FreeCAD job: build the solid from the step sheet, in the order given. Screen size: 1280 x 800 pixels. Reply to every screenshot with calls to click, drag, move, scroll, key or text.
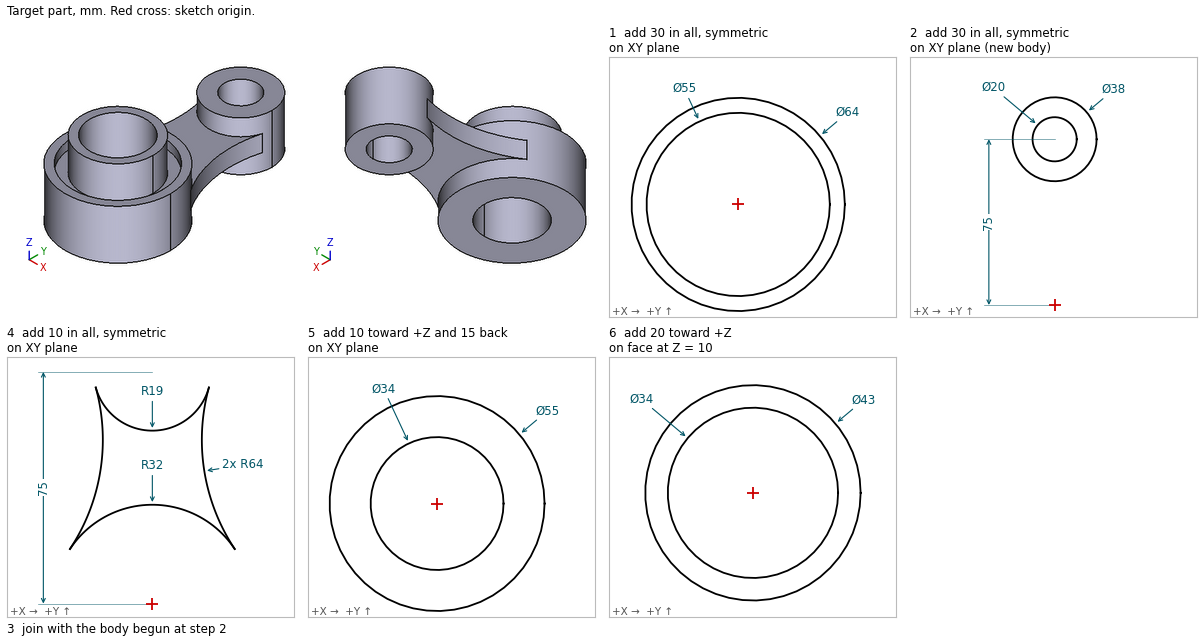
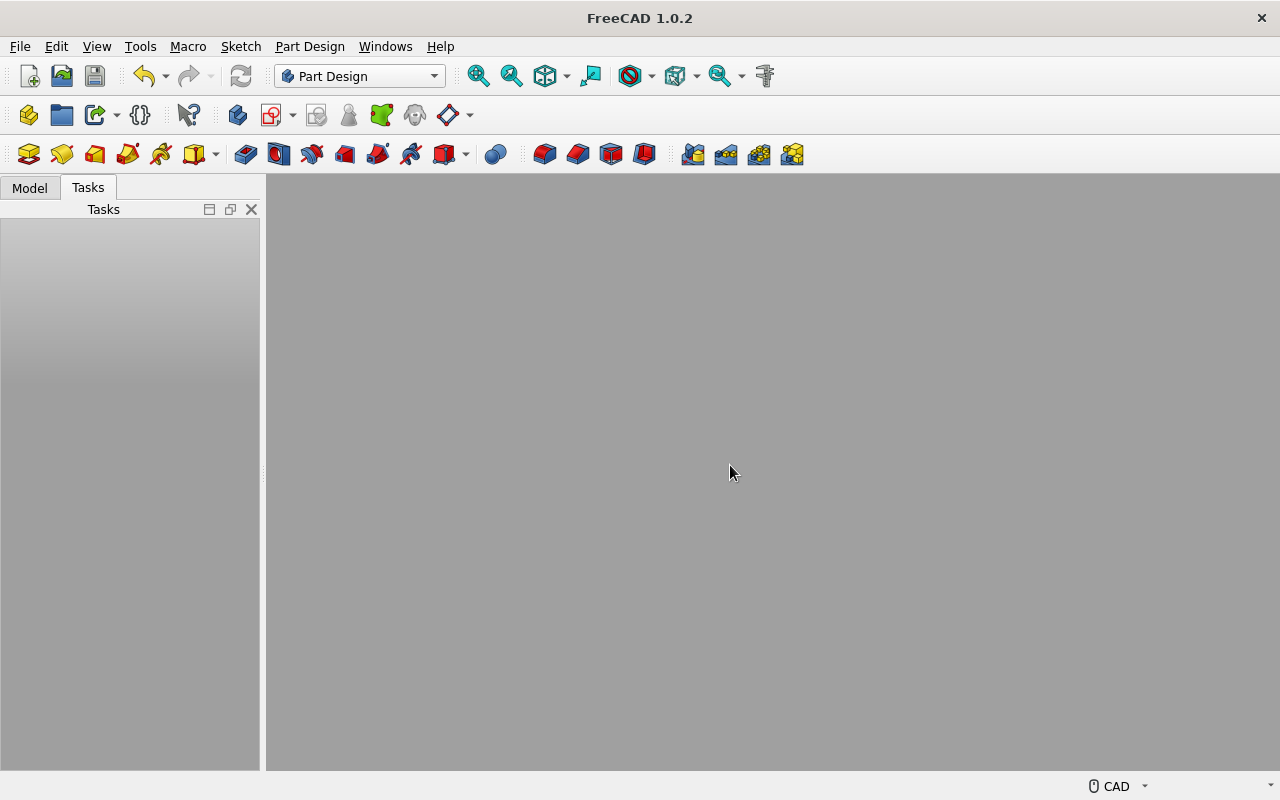
click(29, 76)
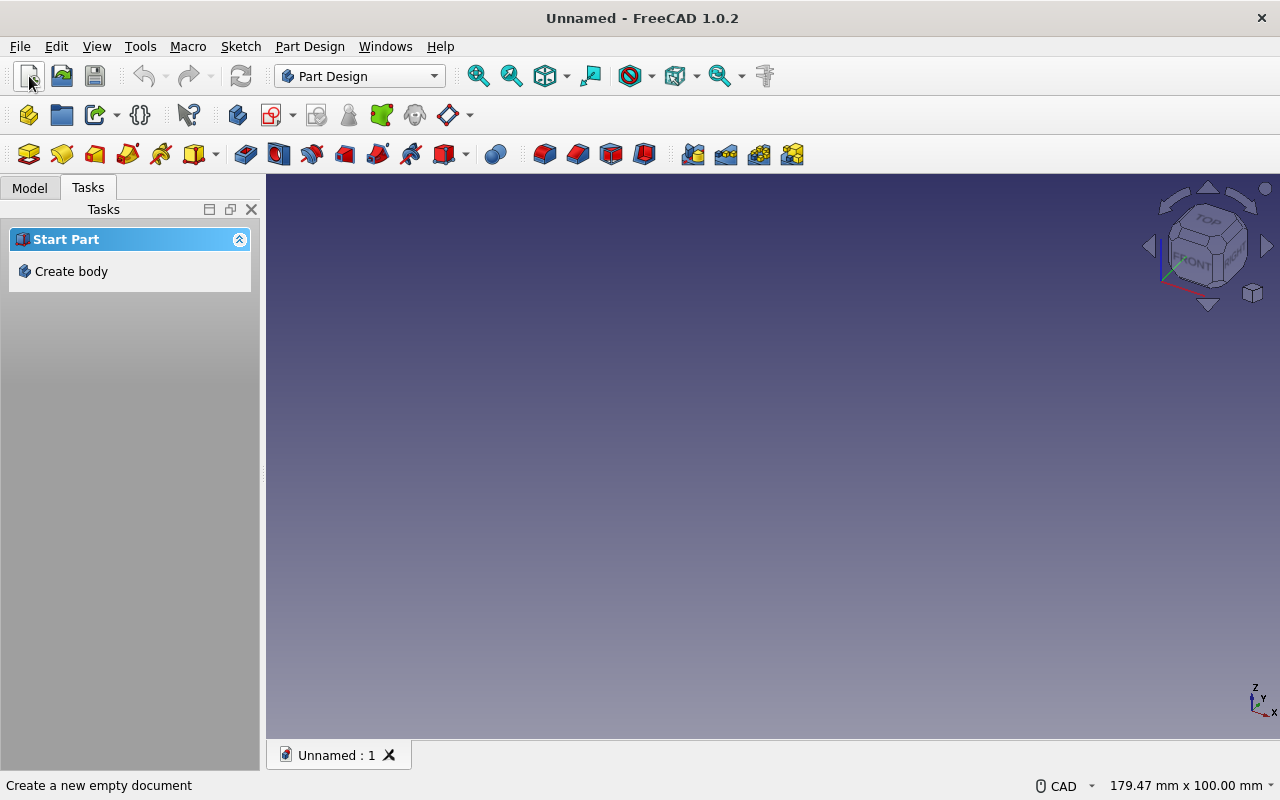
click(270, 116)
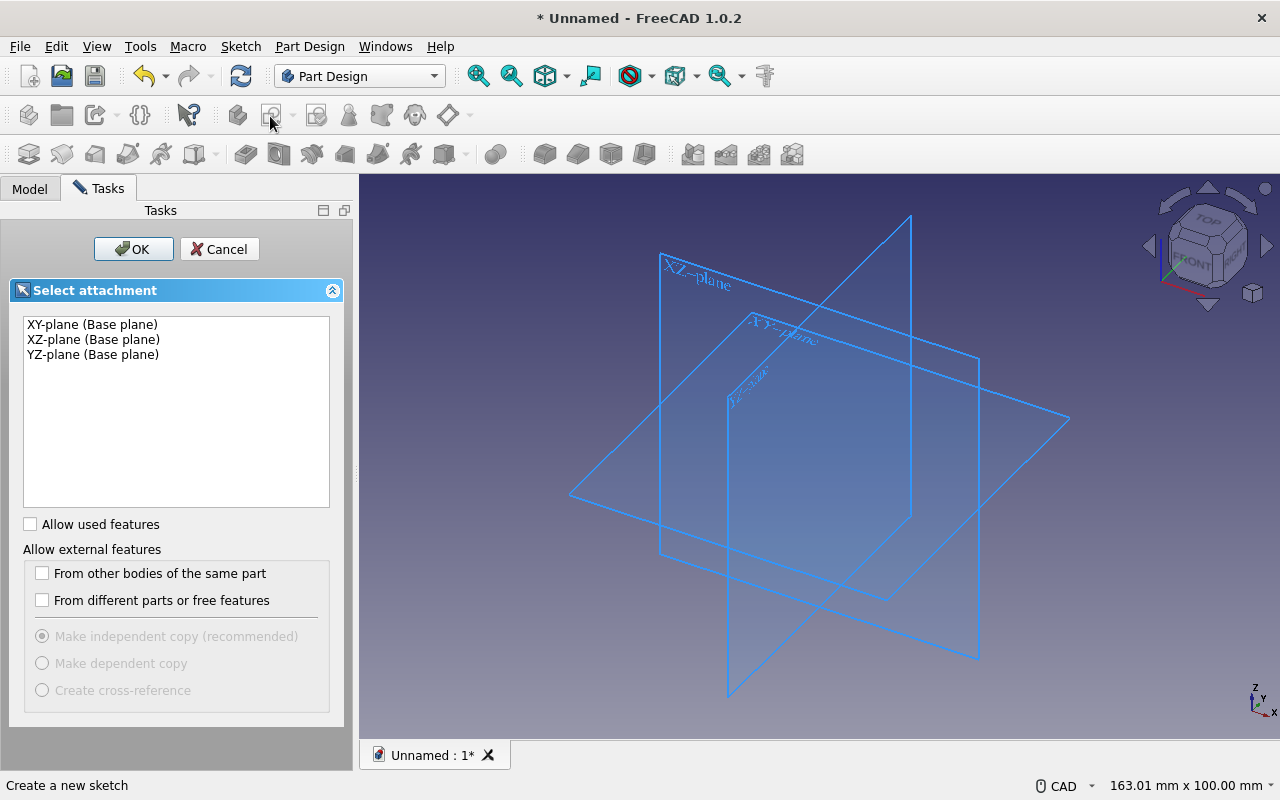
click(84, 324)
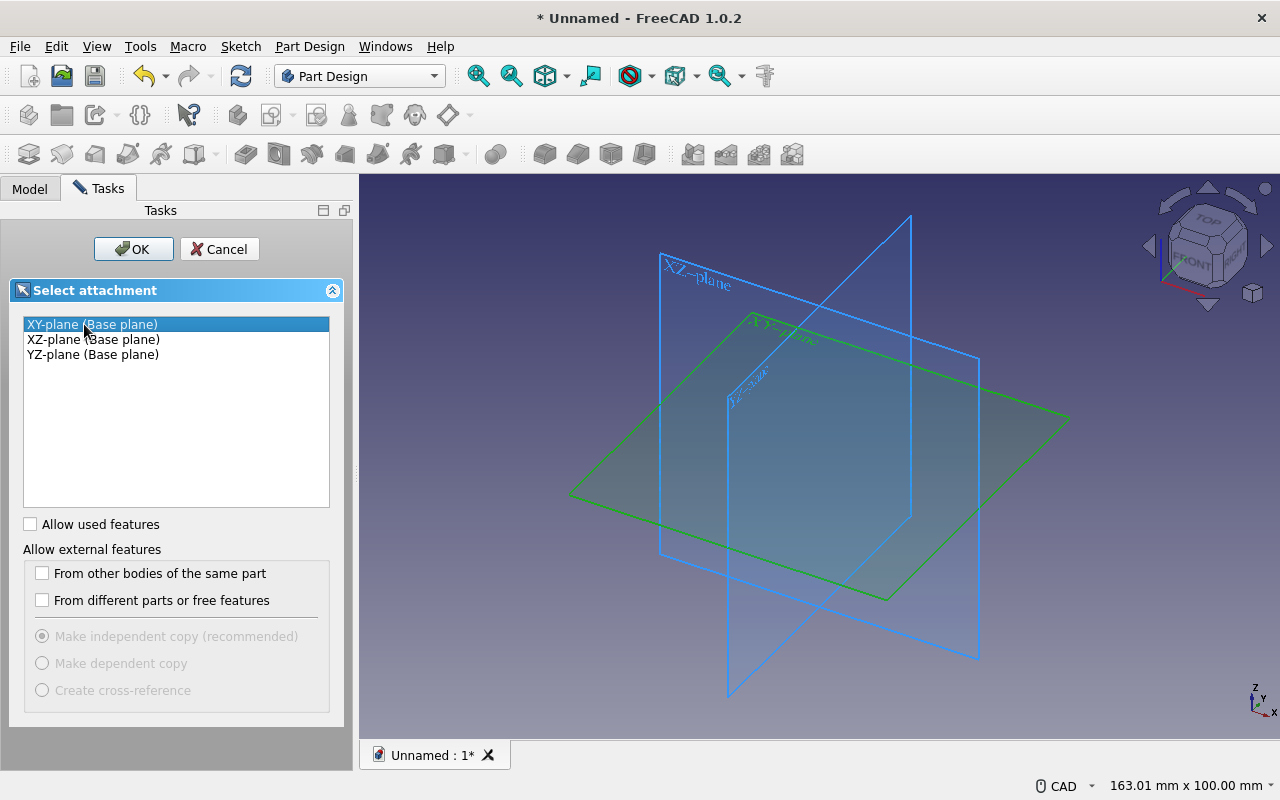
click(134, 249)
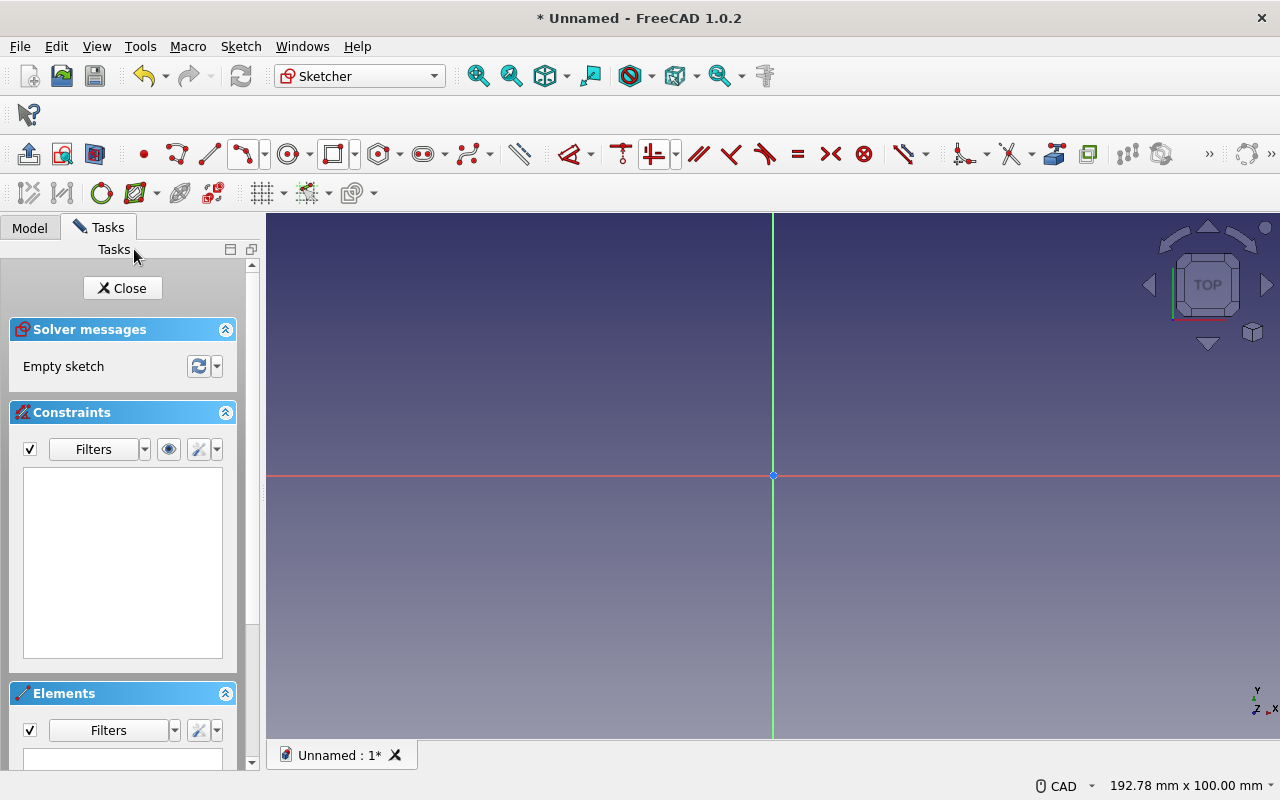
key(g)
key(c)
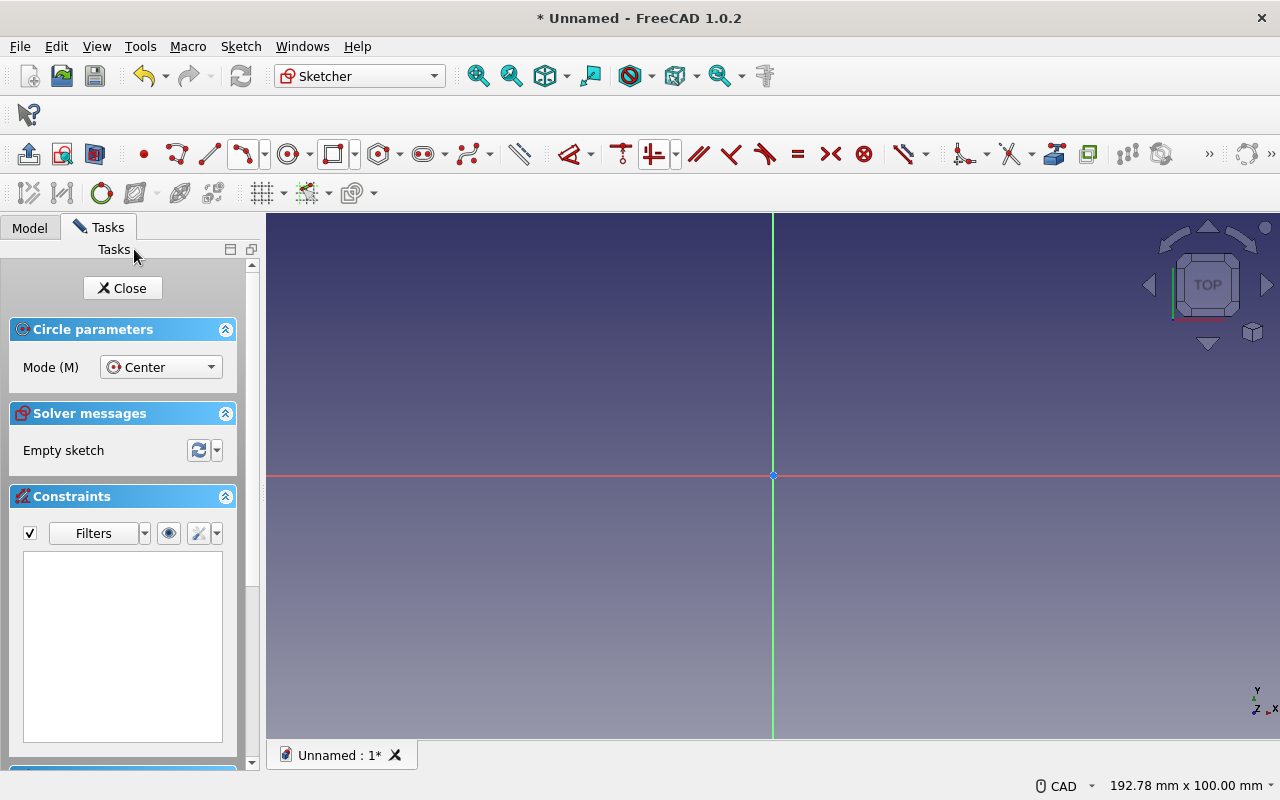
click(773, 476)
click(892, 357)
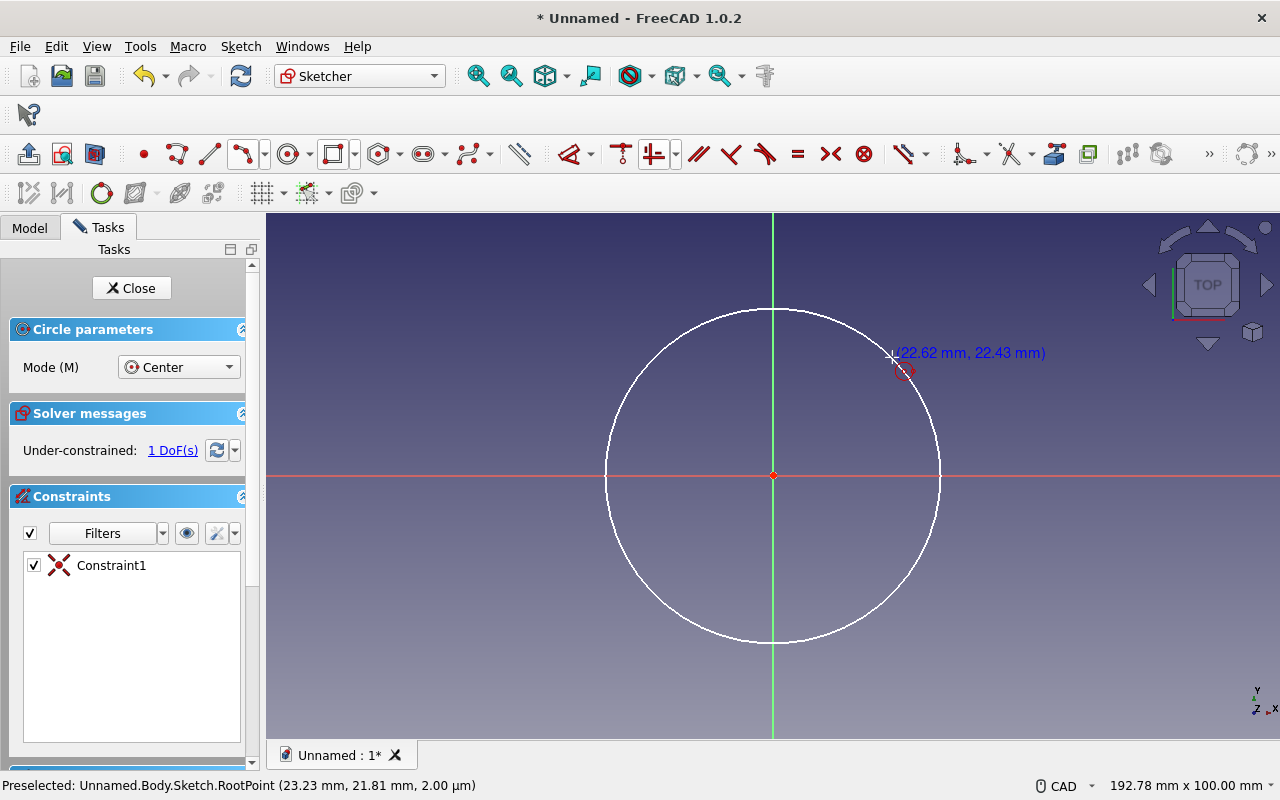
click(773, 476)
click(875, 374)
key(Escape)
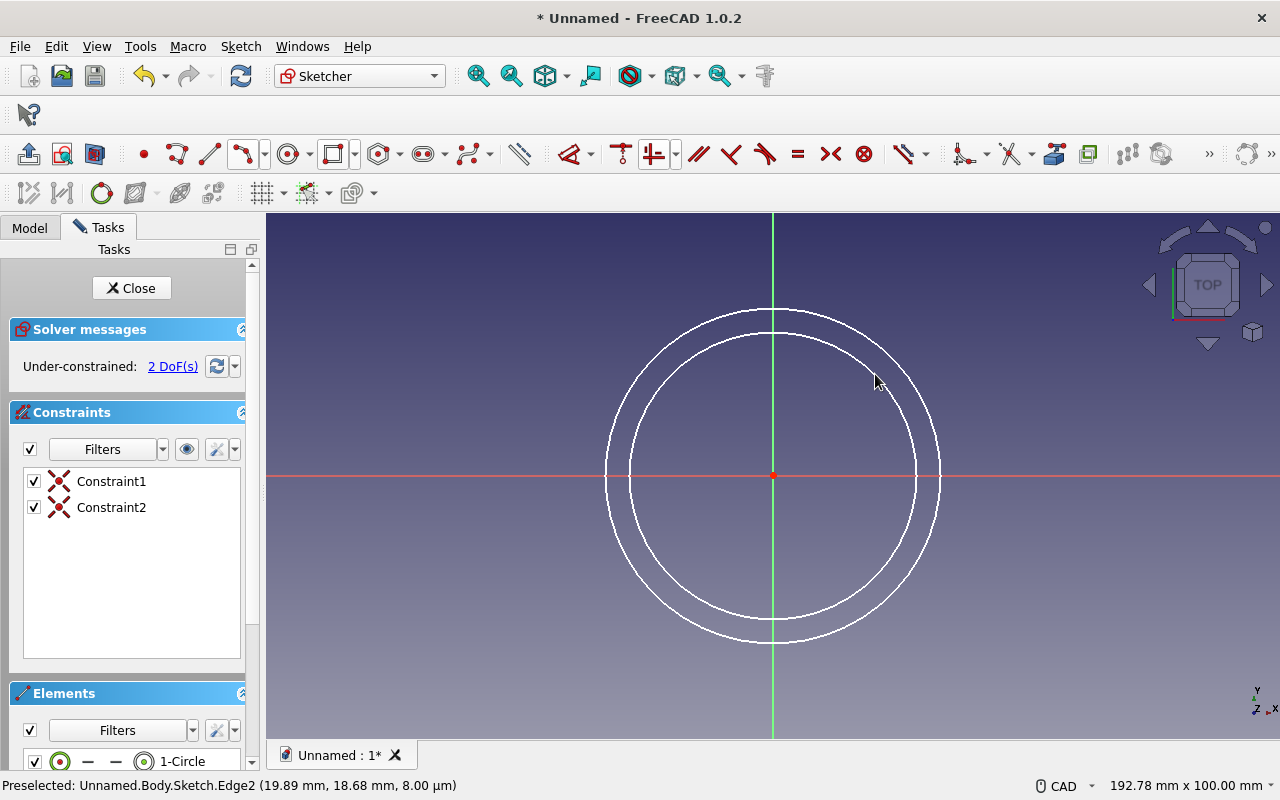
key(d)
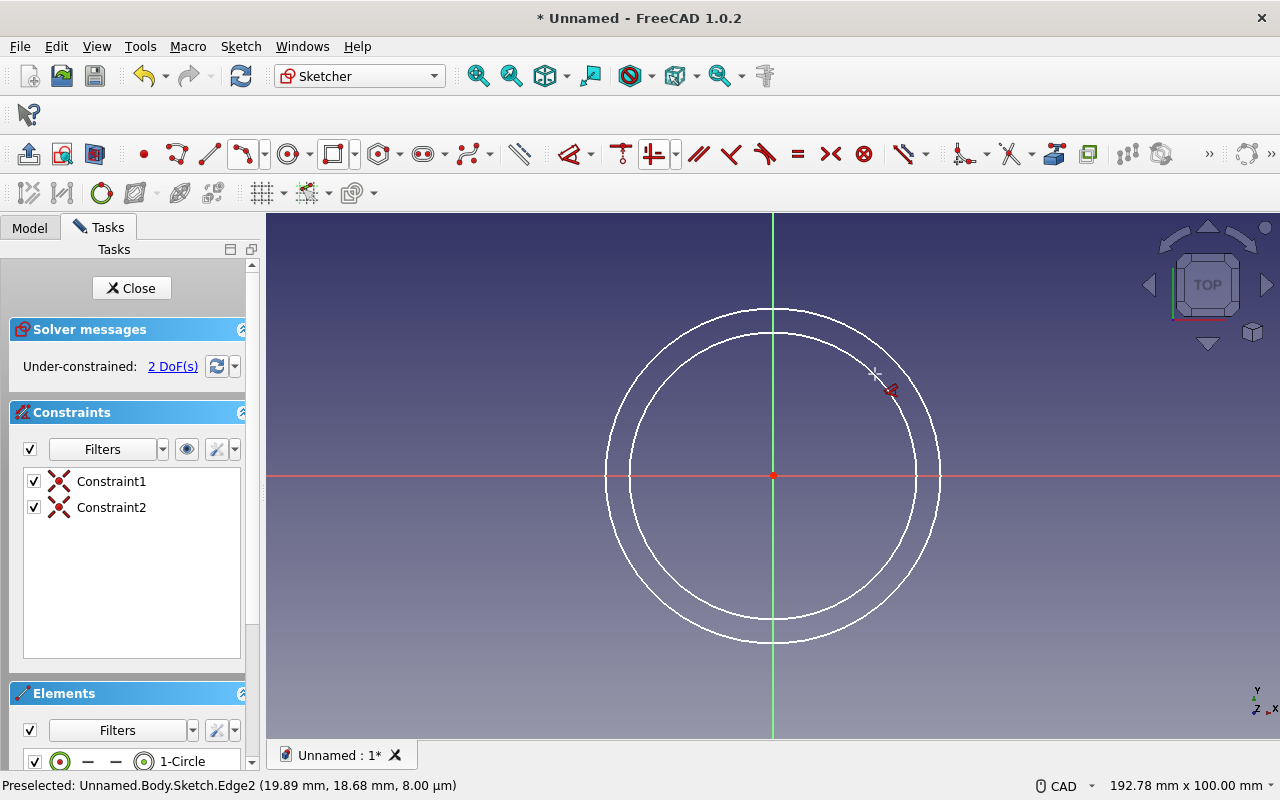
click(891, 357)
click(914, 334)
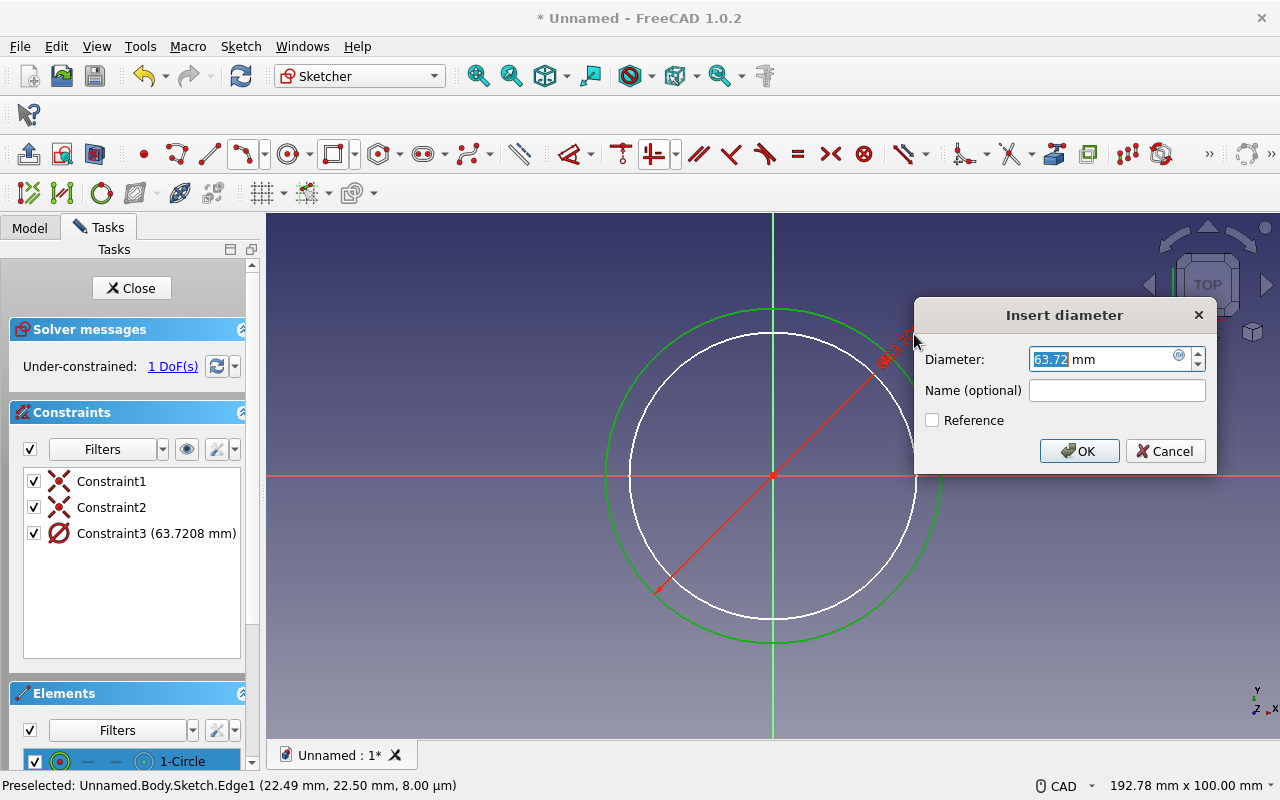
text(64)
key(Return)